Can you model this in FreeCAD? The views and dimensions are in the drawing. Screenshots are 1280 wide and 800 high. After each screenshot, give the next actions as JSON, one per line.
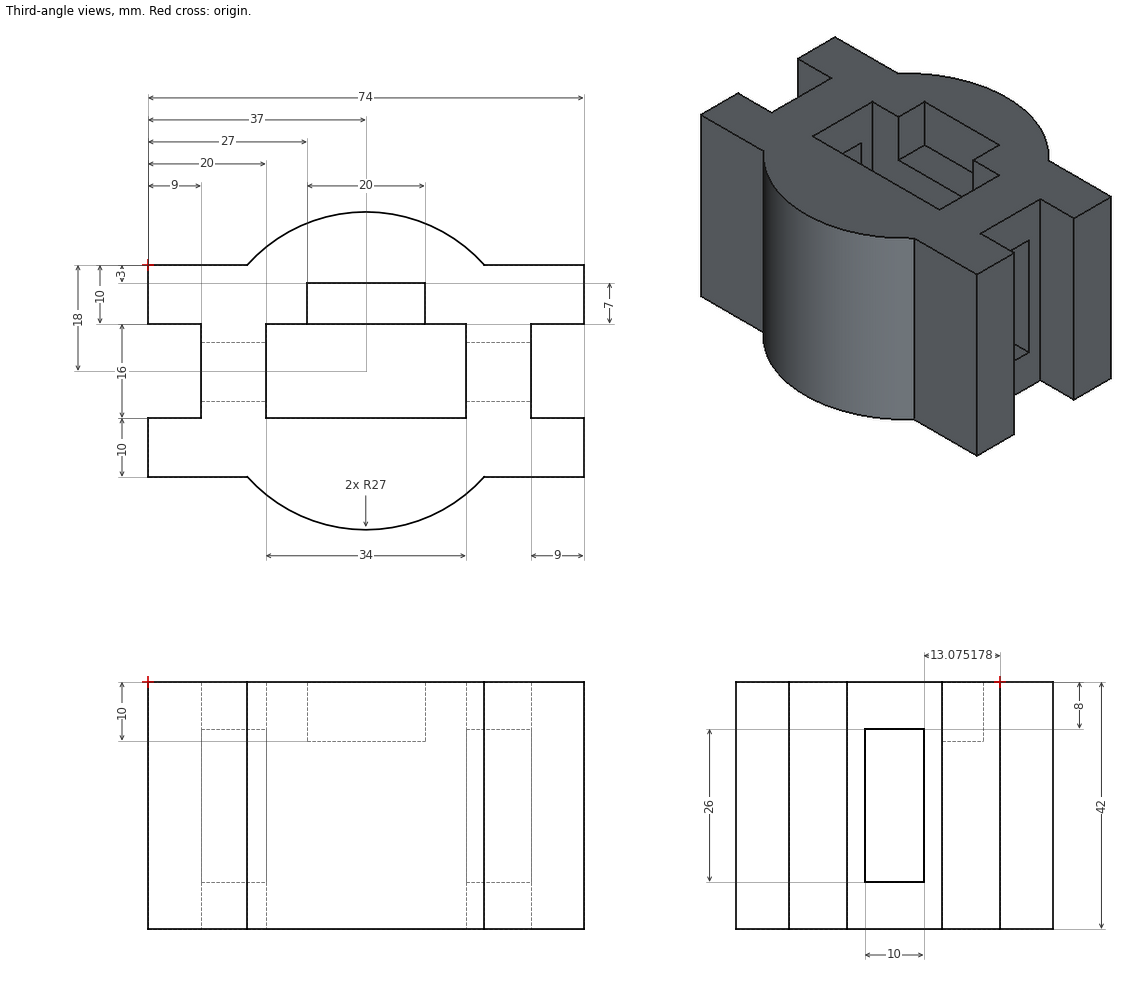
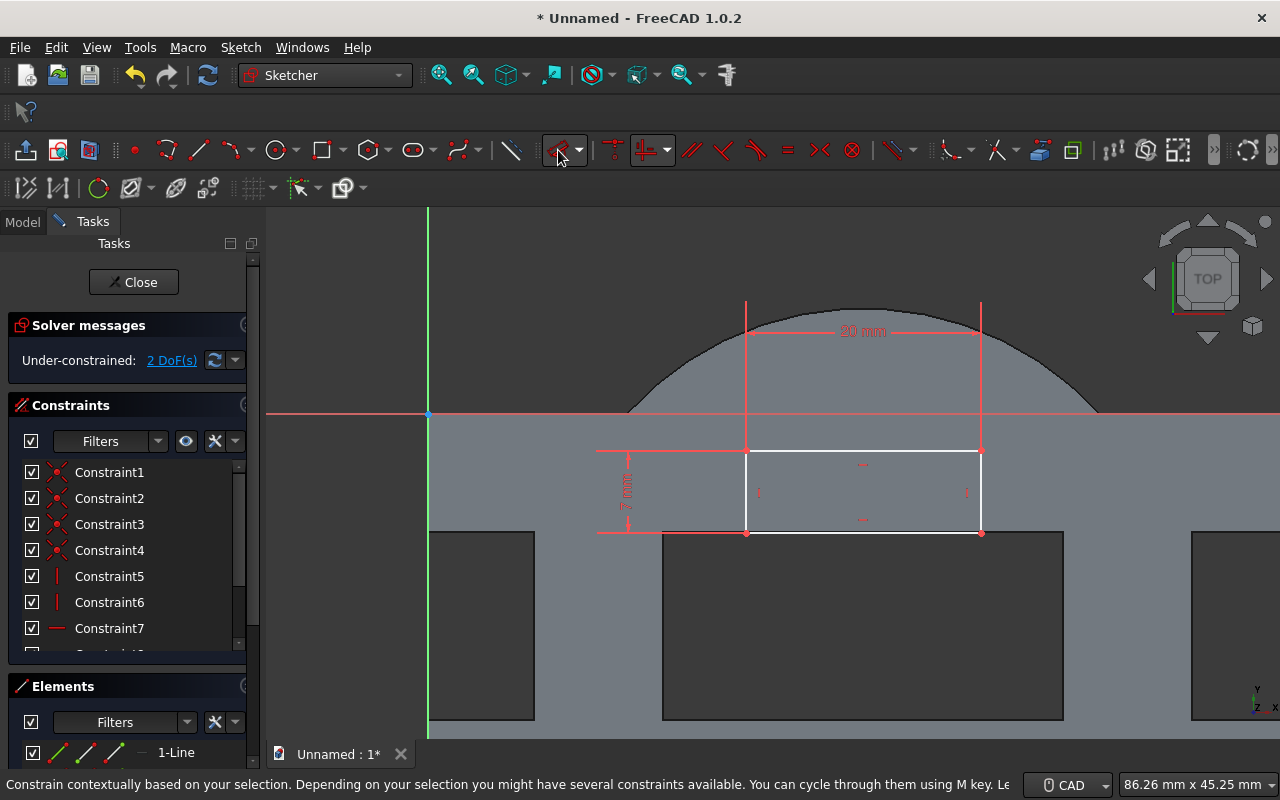
{"action": "left_click", "coordinate": [746, 451]}
{"action": "left_click", "coordinate": [394, 433]}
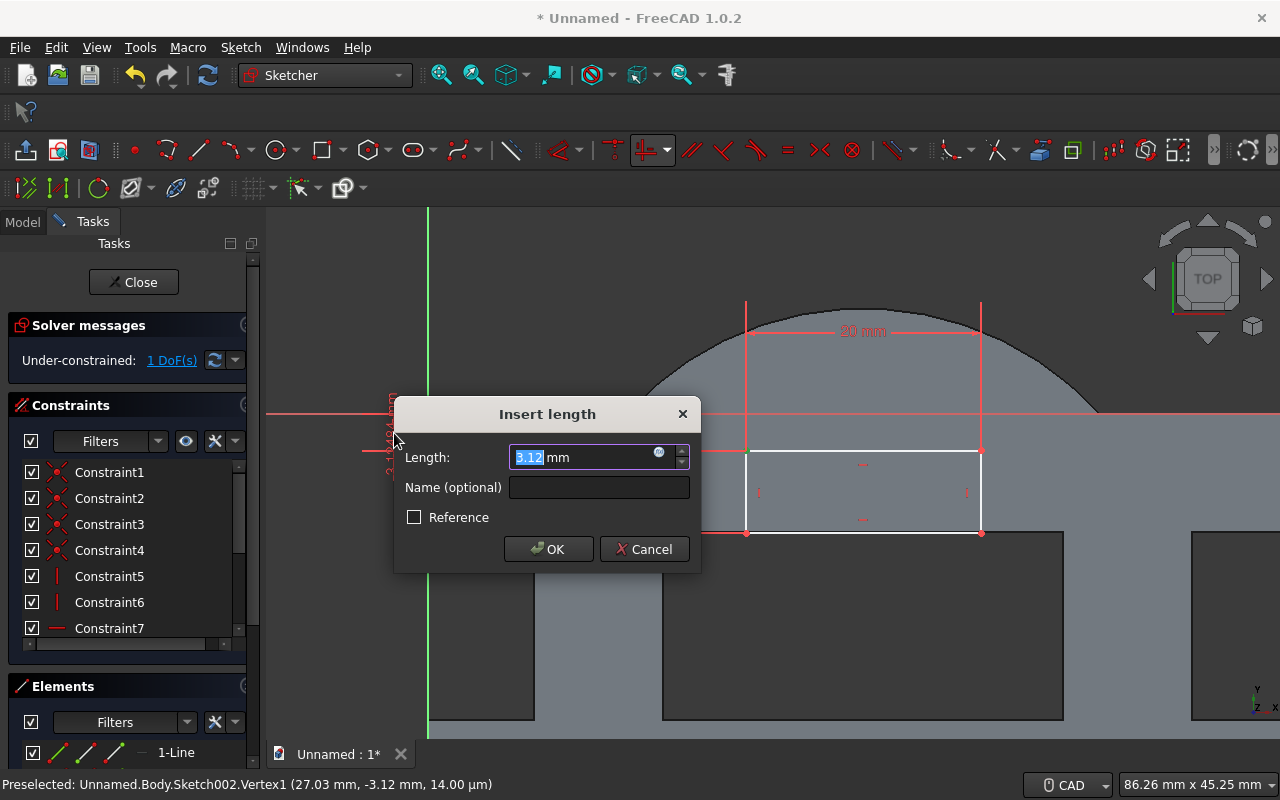
{"action": "type", "text": "3"}
{"action": "key", "text": "Return"}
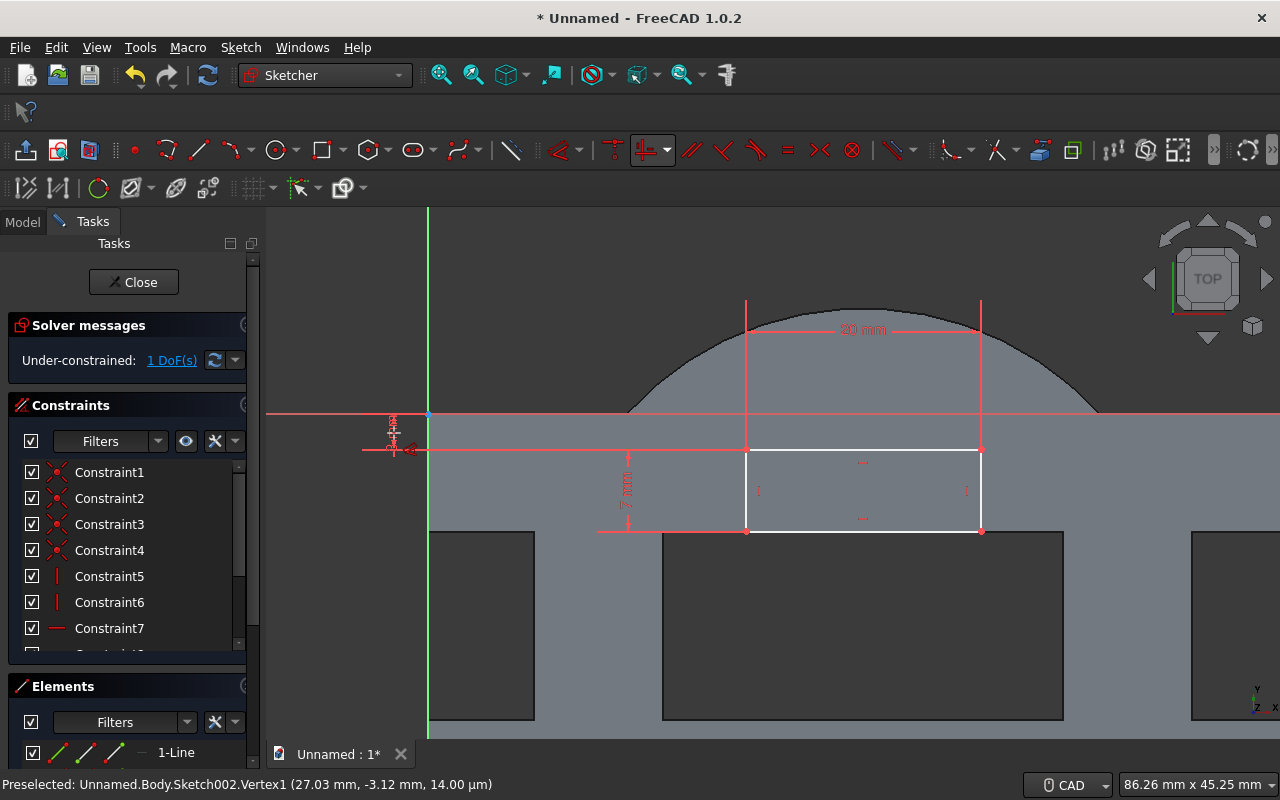
{"action": "left_click", "coordinate": [746, 450]}
{"action": "left_click", "coordinate": [587, 380]}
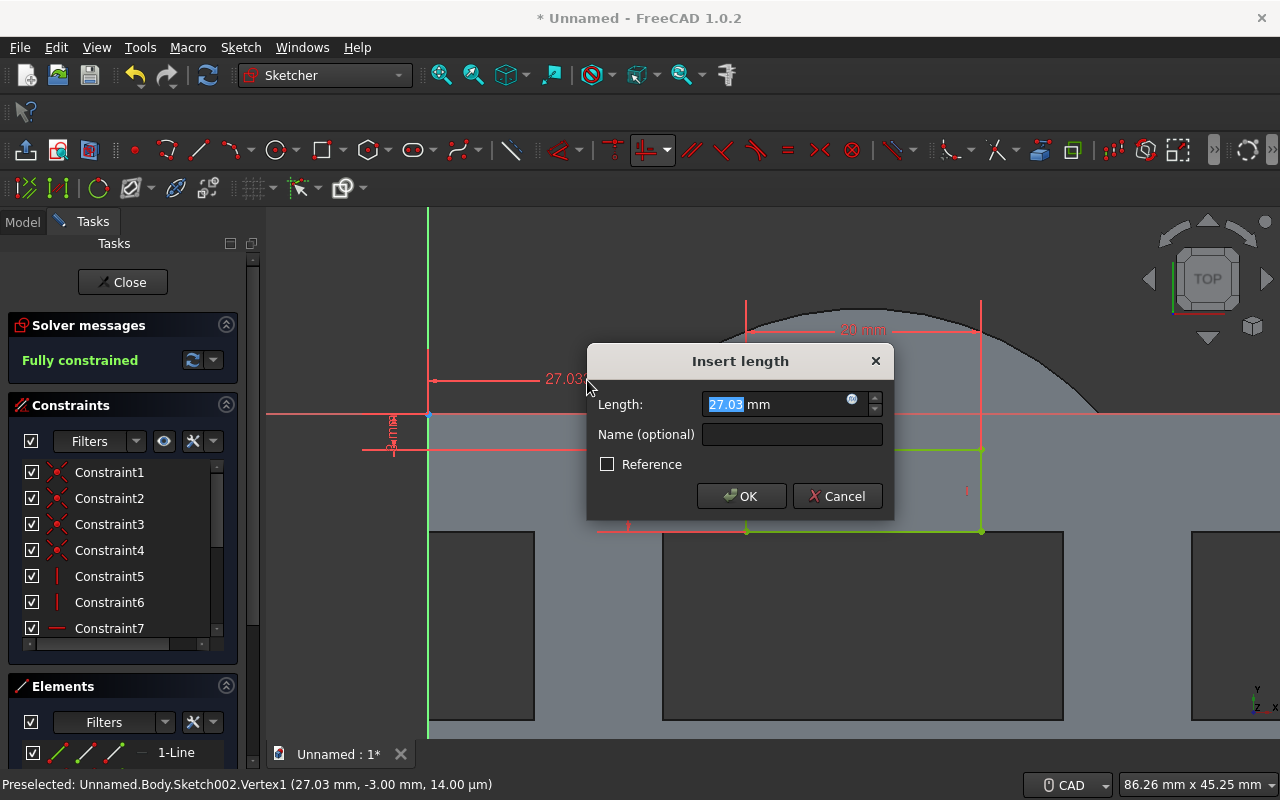
{"action": "type", "text": "27"}
{"action": "key", "text": "Return"}
{"action": "key", "text": "Escape"}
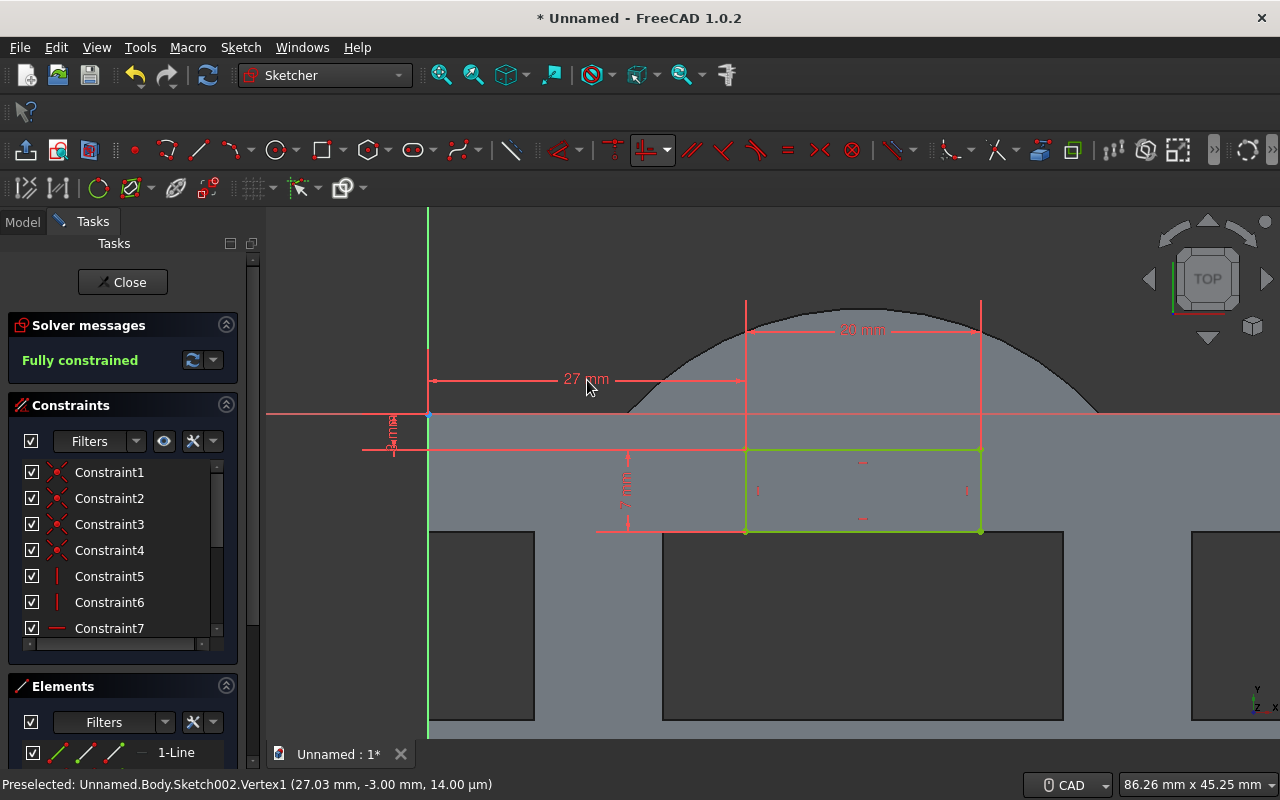
{"action": "left_click", "coordinate": [123, 282]}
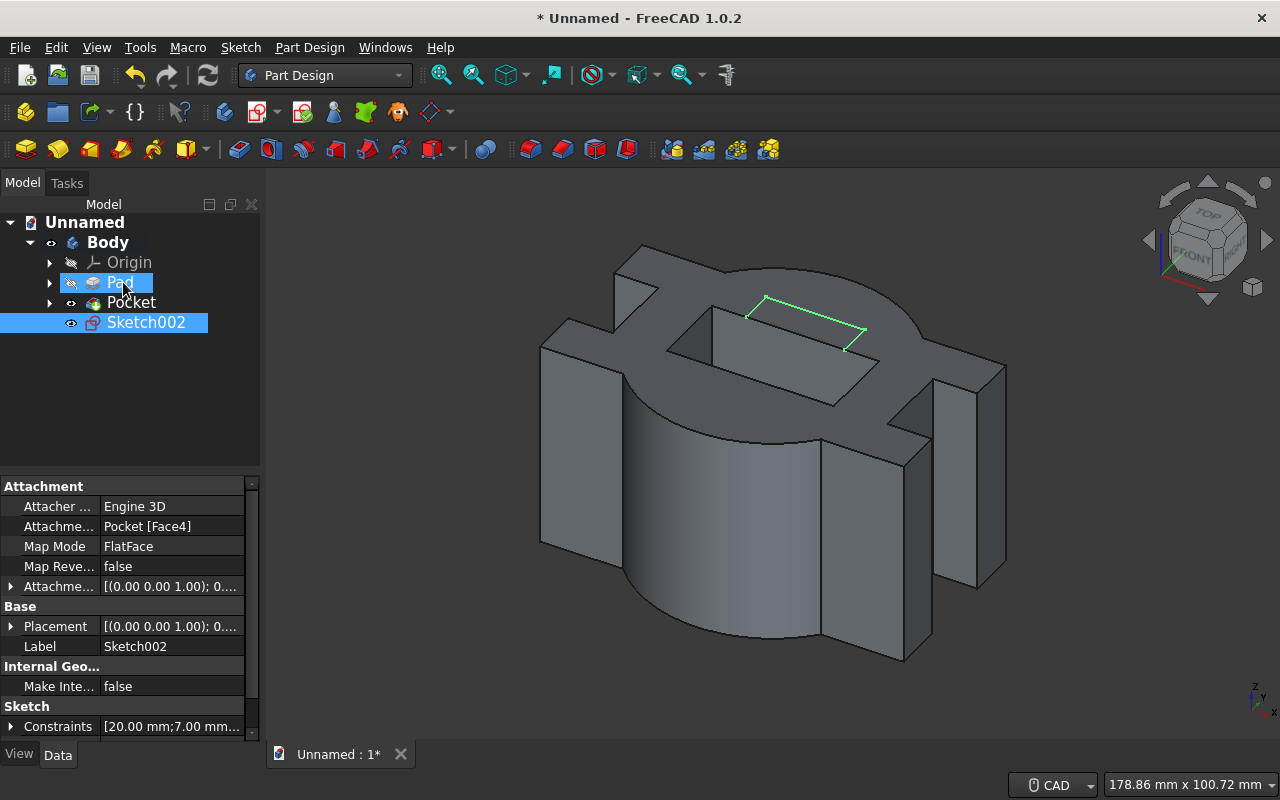
{"action": "left_click", "coordinate": [240, 150]}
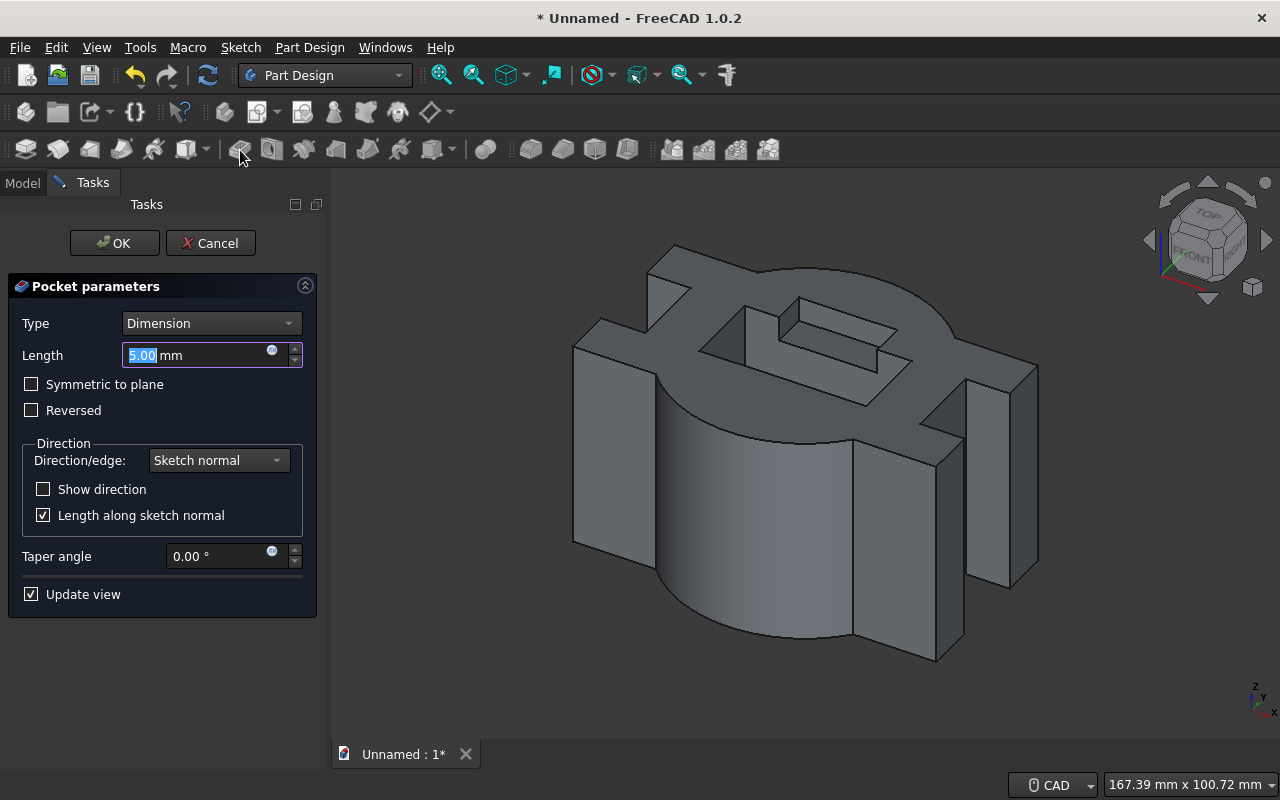
{"action": "type", "text": "10"}
{"action": "key", "text": "Tab"}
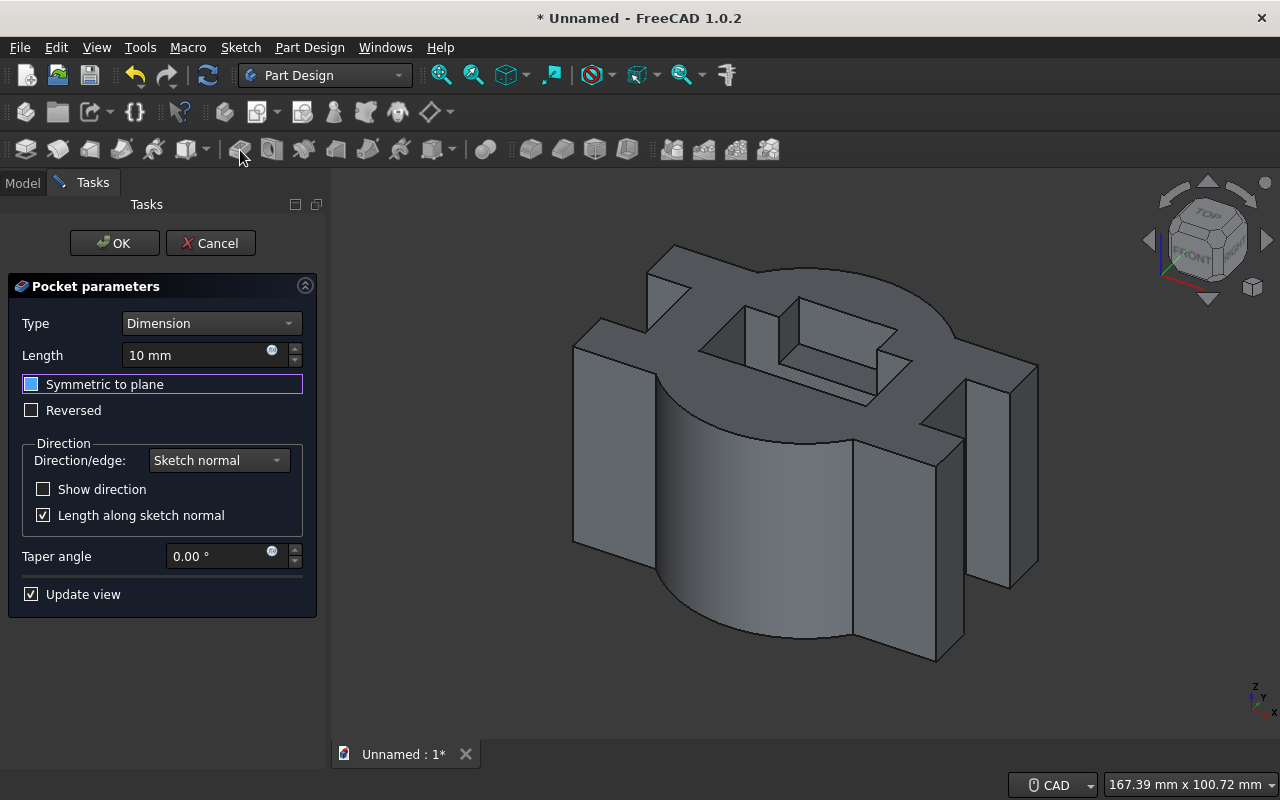
{"action": "left_click", "coordinate": [115, 243]}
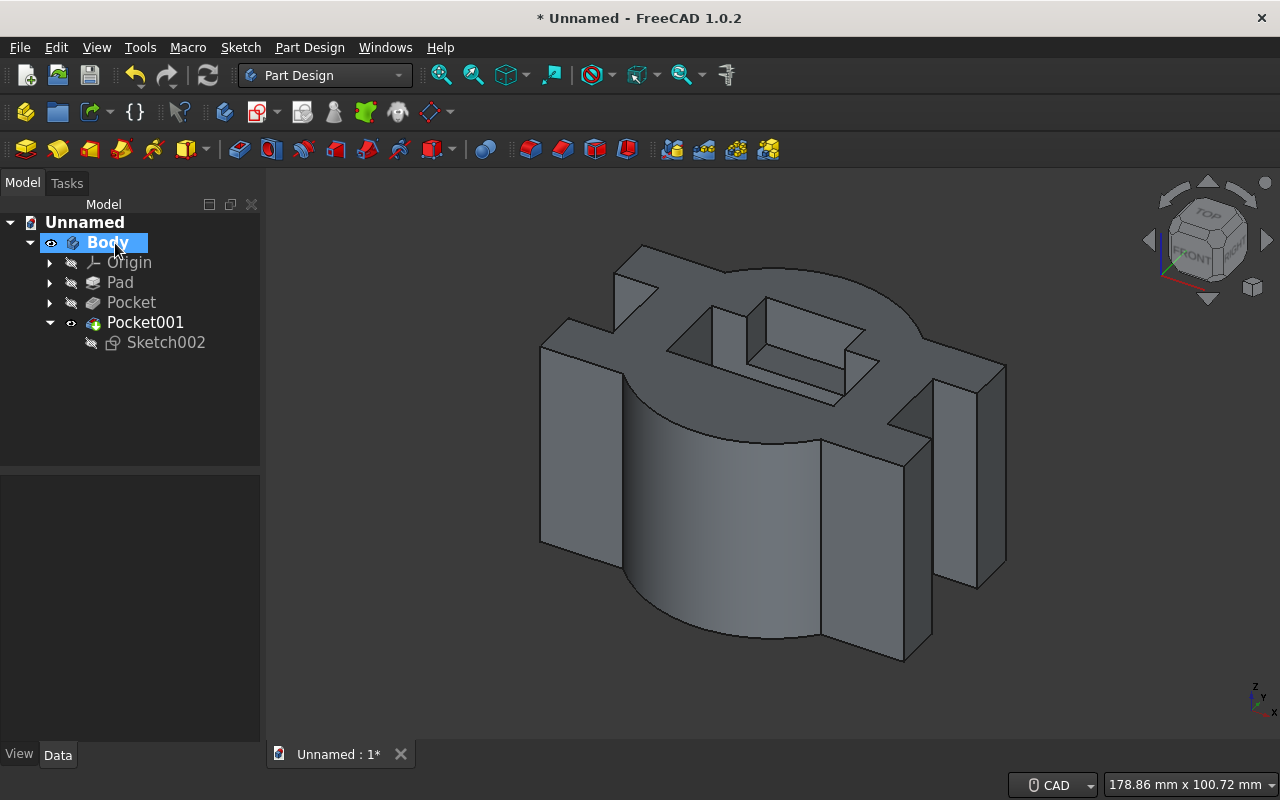
{"action": "key", "text": "6"}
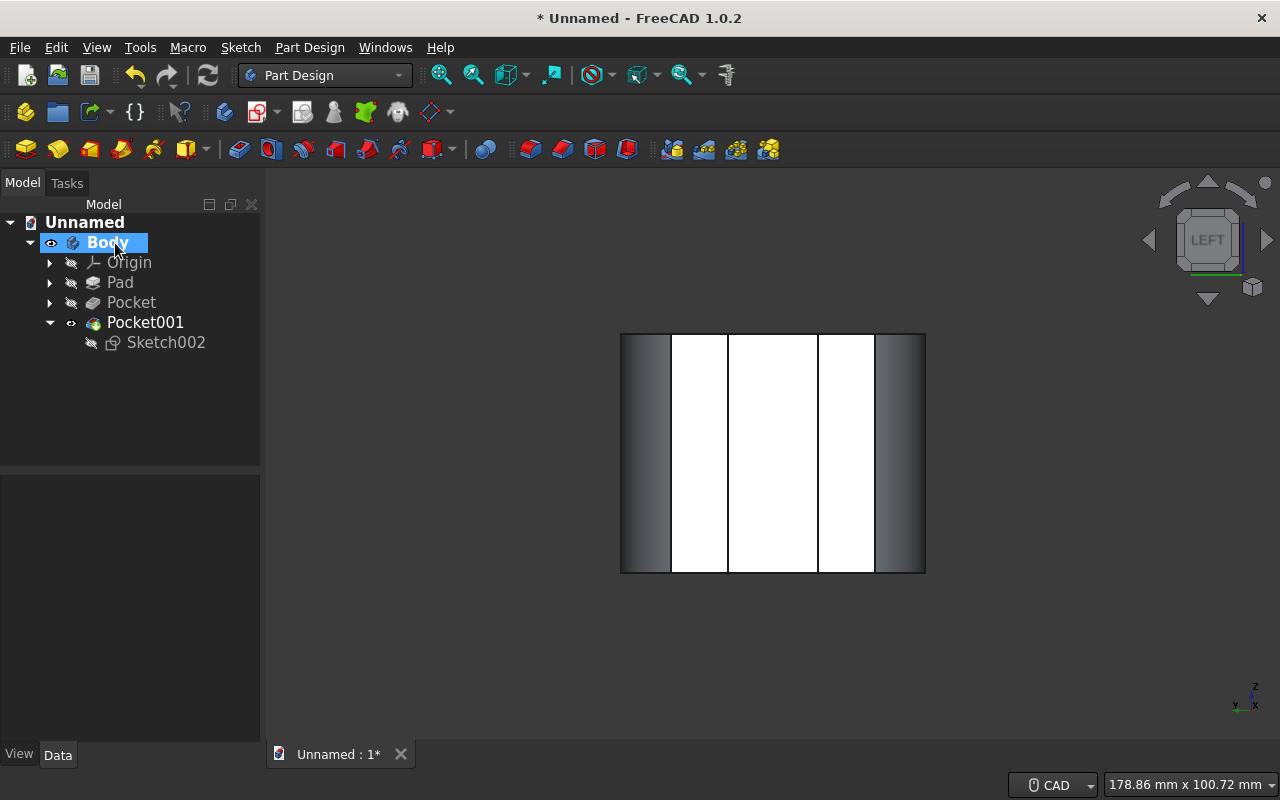
{"action": "left_click", "coordinate": [442, 76]}